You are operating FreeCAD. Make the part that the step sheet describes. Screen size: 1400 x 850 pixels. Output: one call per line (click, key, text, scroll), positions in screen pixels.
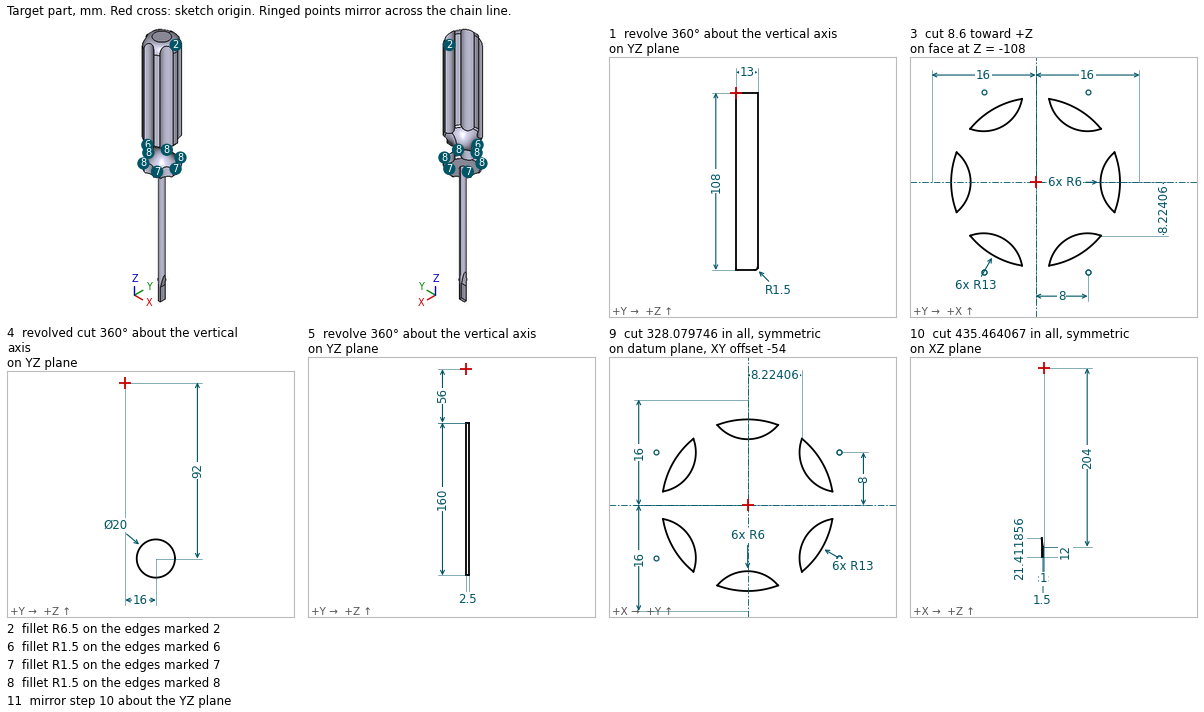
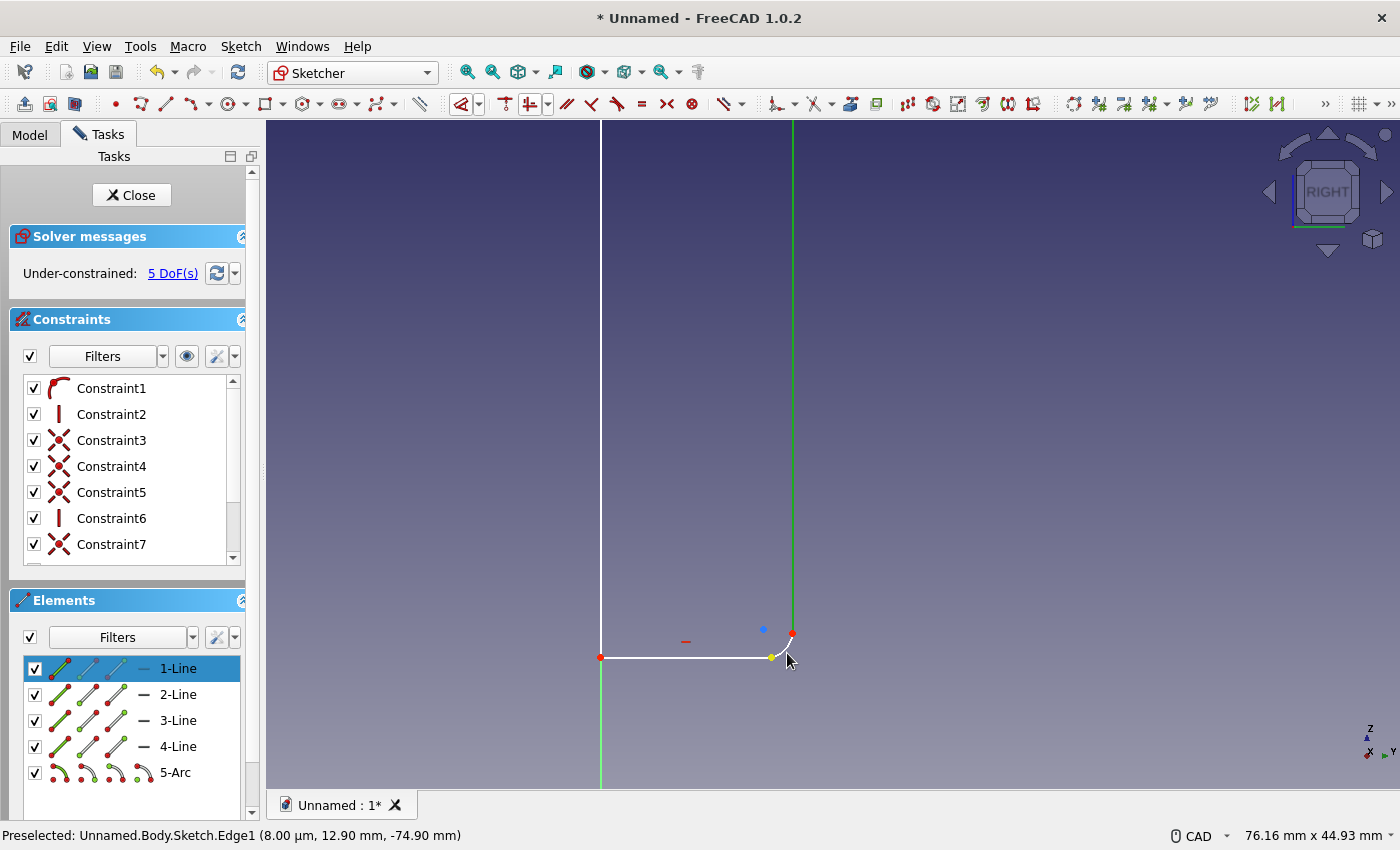
click(786, 649)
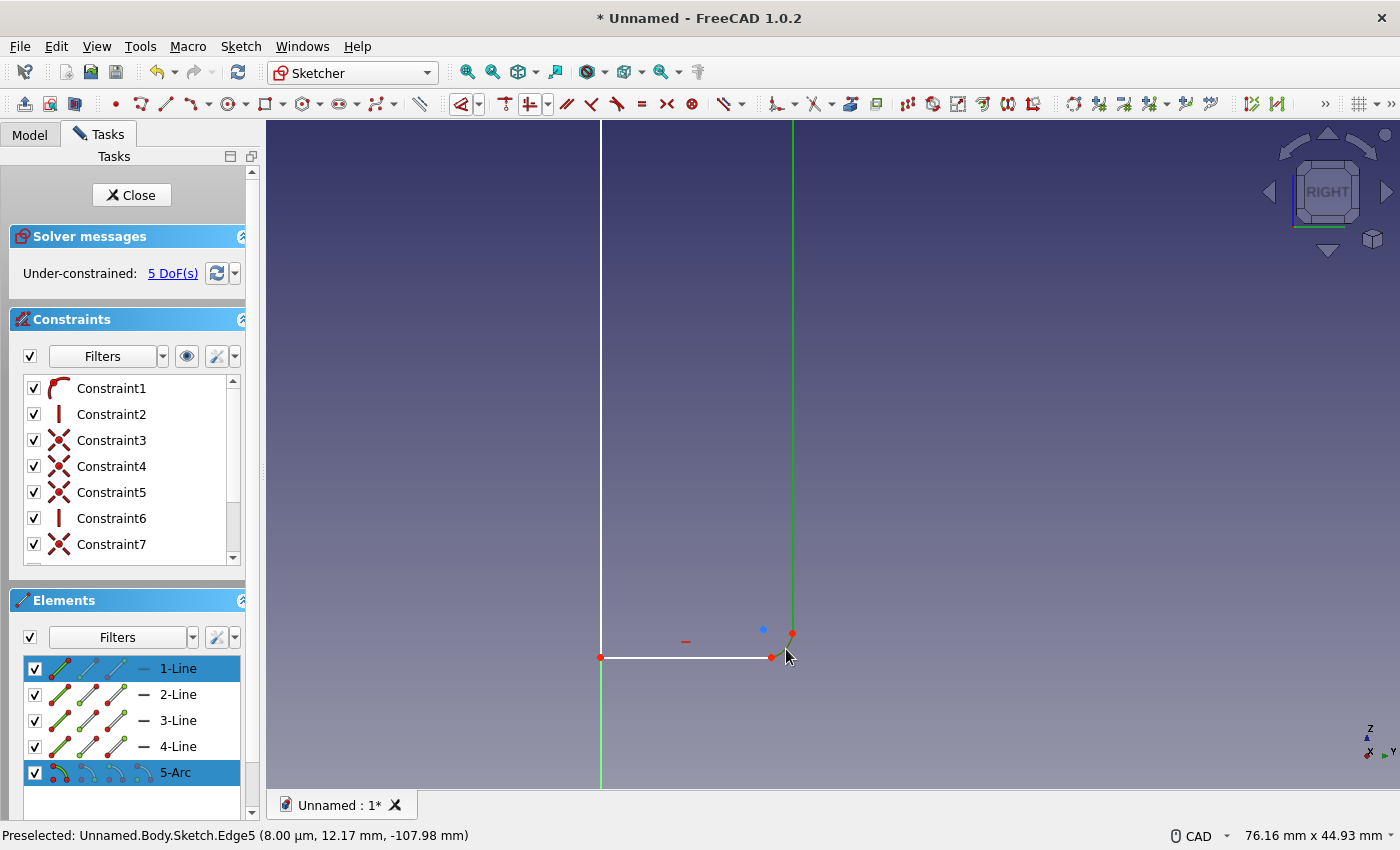
key(t)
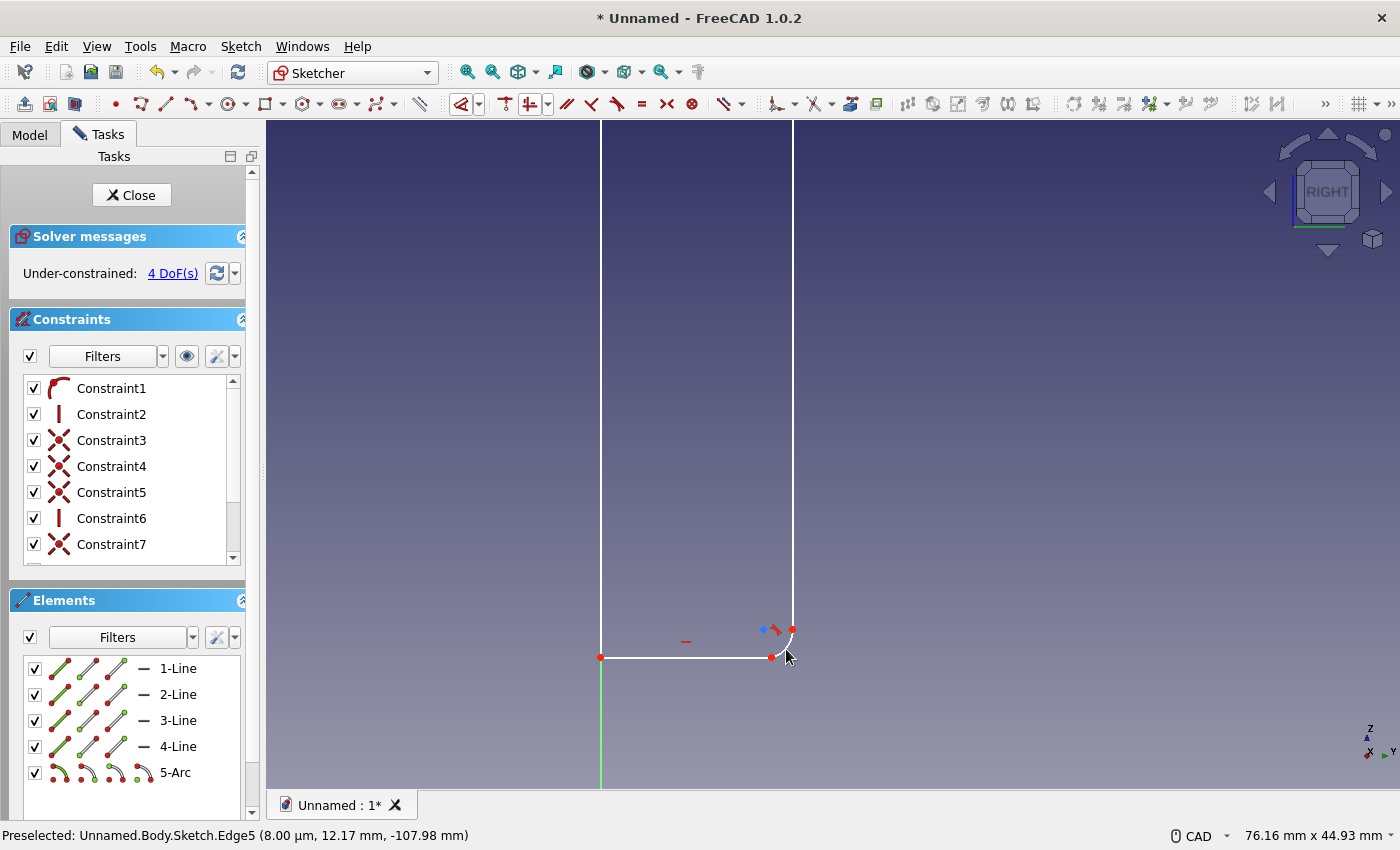
scroll(786, 653, down, 7)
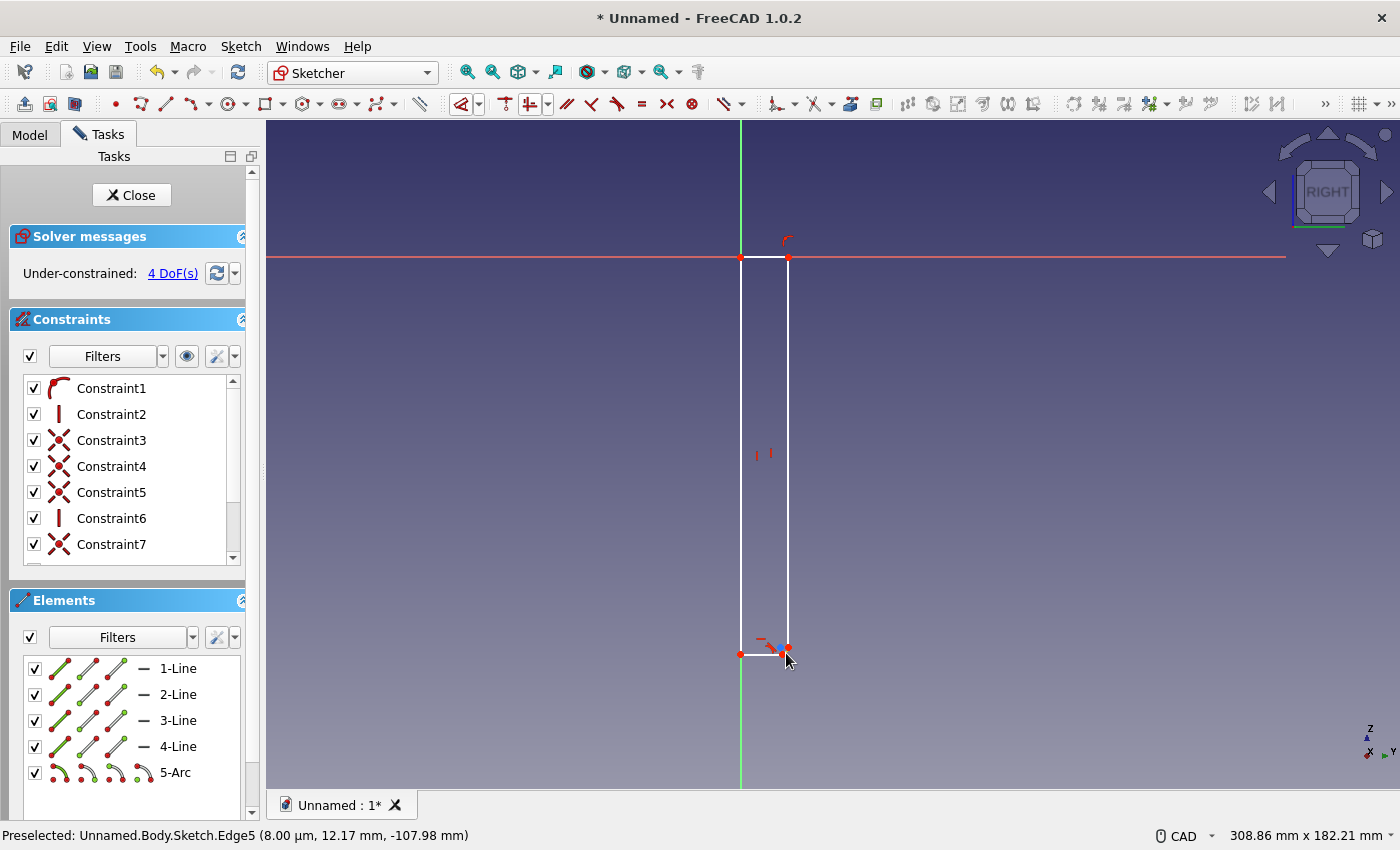
click(753, 655)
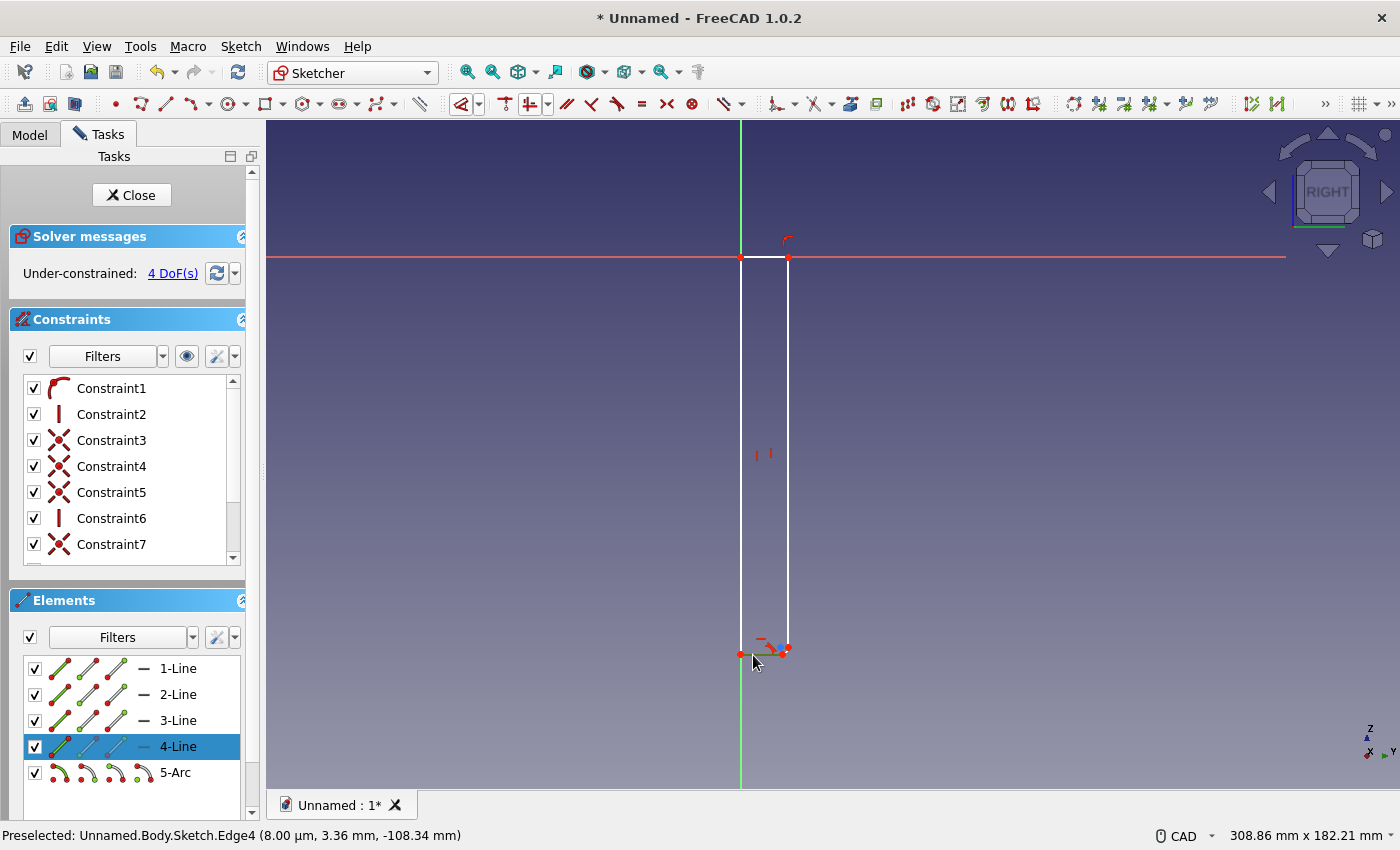
scroll(787, 652, up, 6)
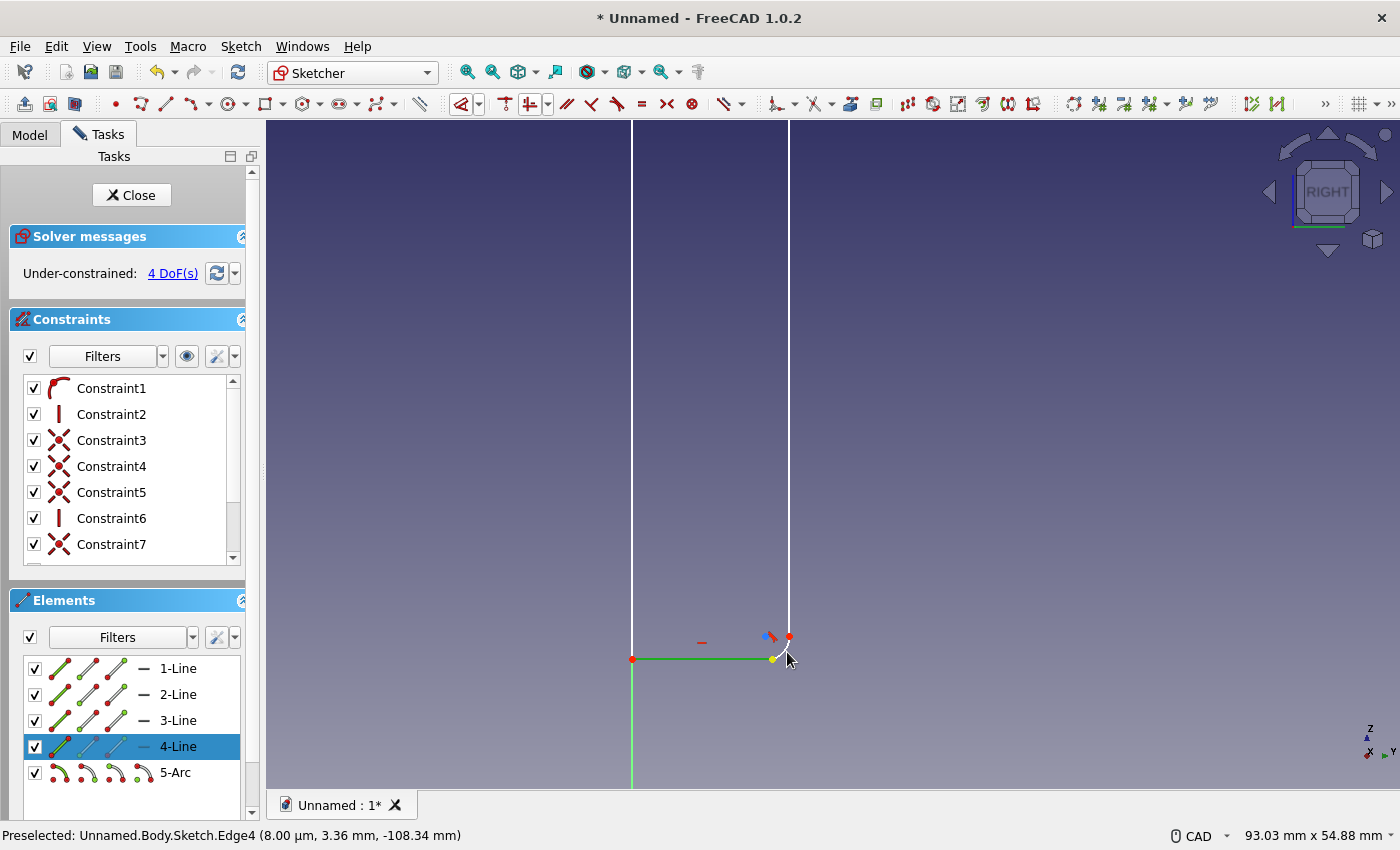
click(785, 651)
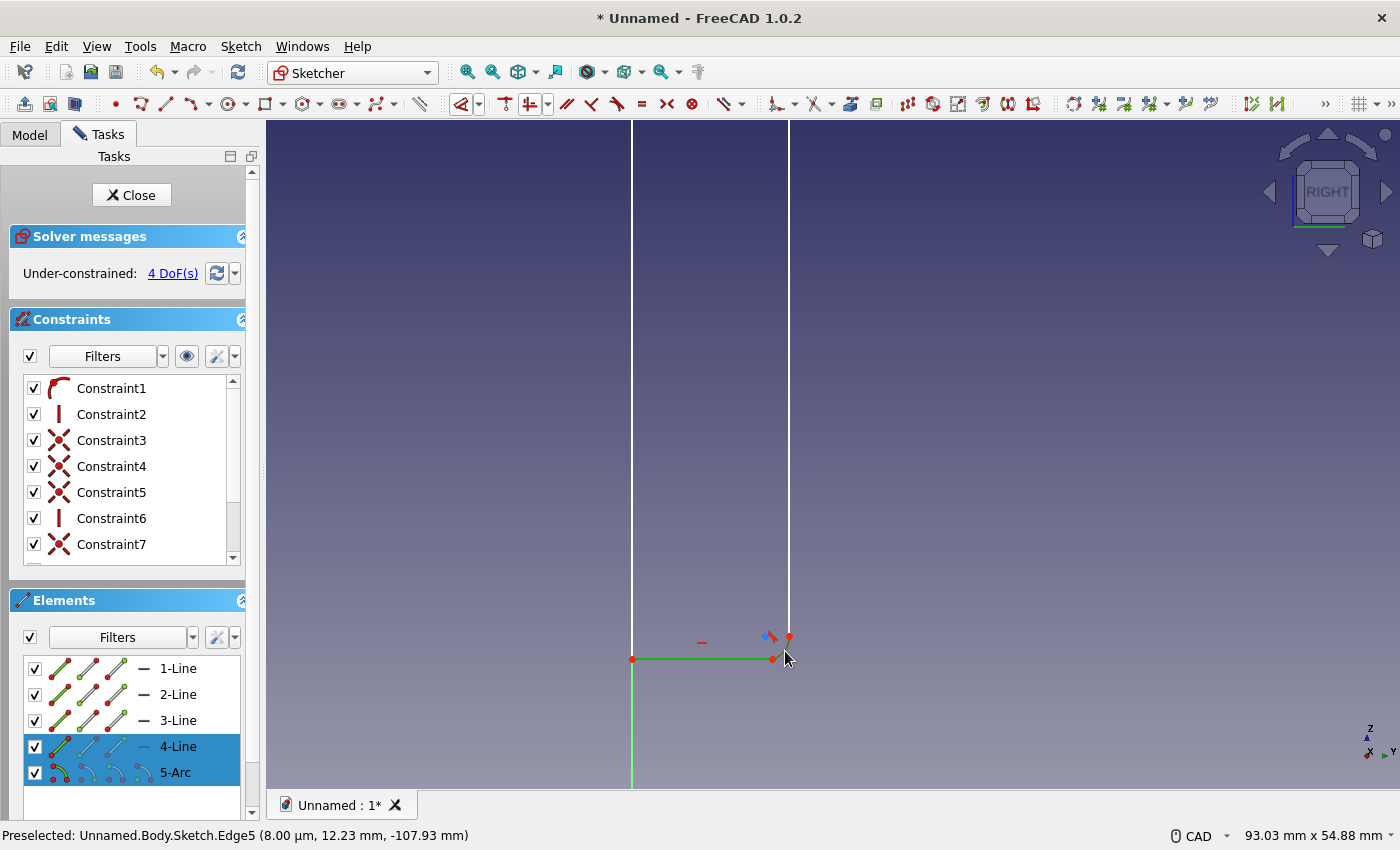
key(t)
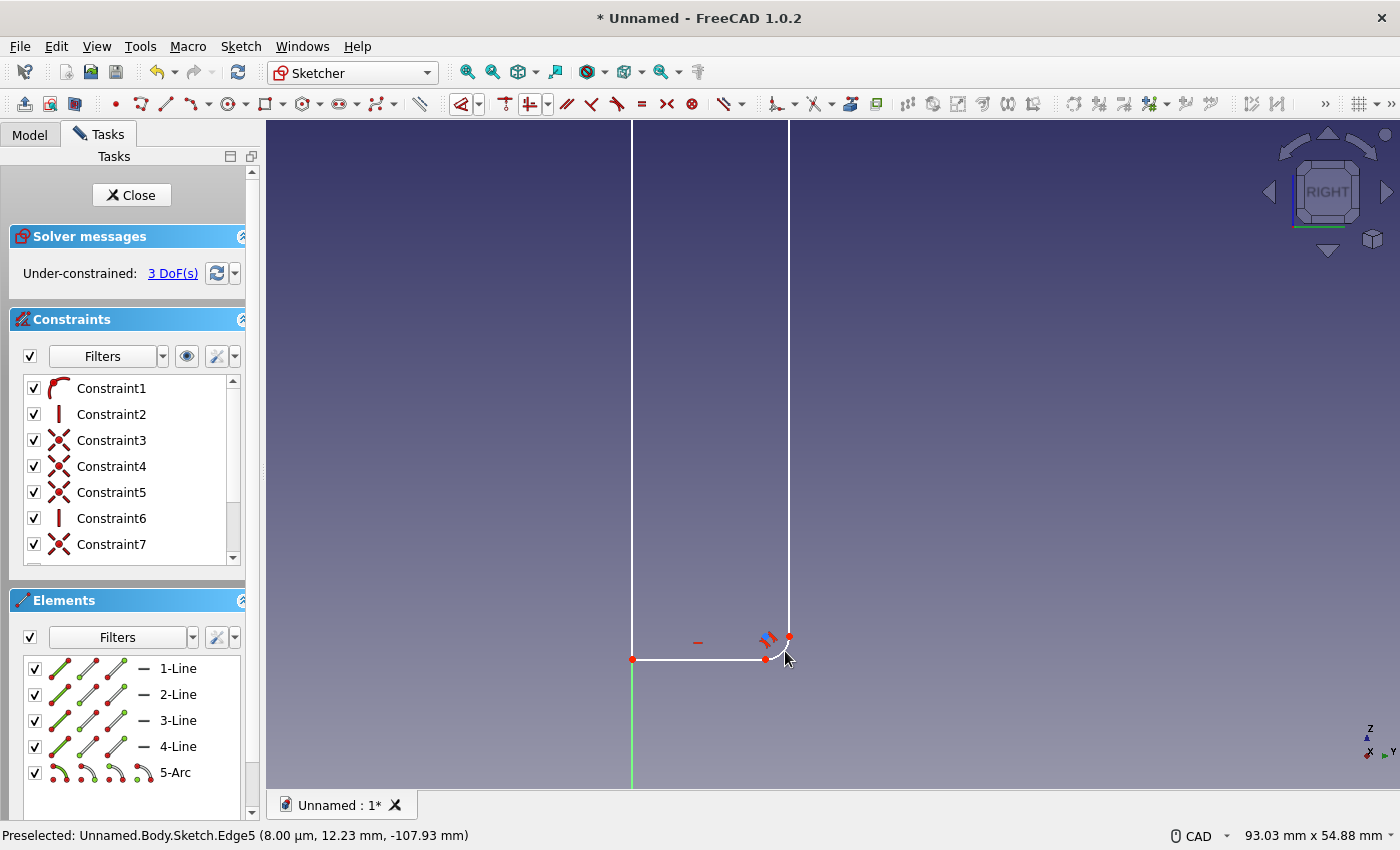
key(d)